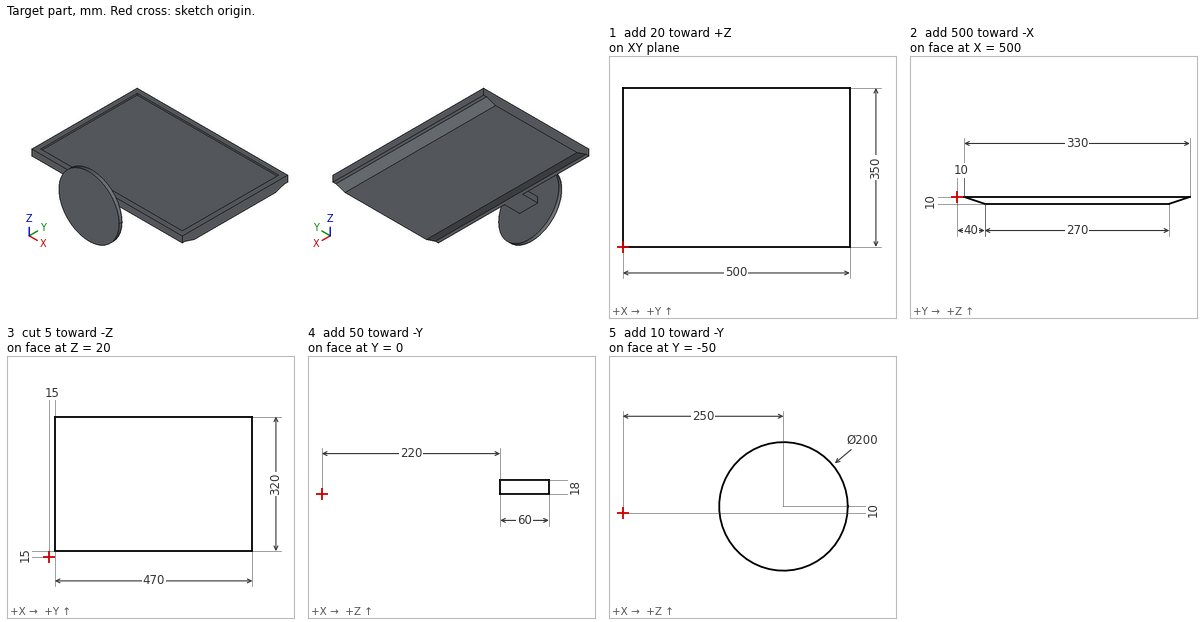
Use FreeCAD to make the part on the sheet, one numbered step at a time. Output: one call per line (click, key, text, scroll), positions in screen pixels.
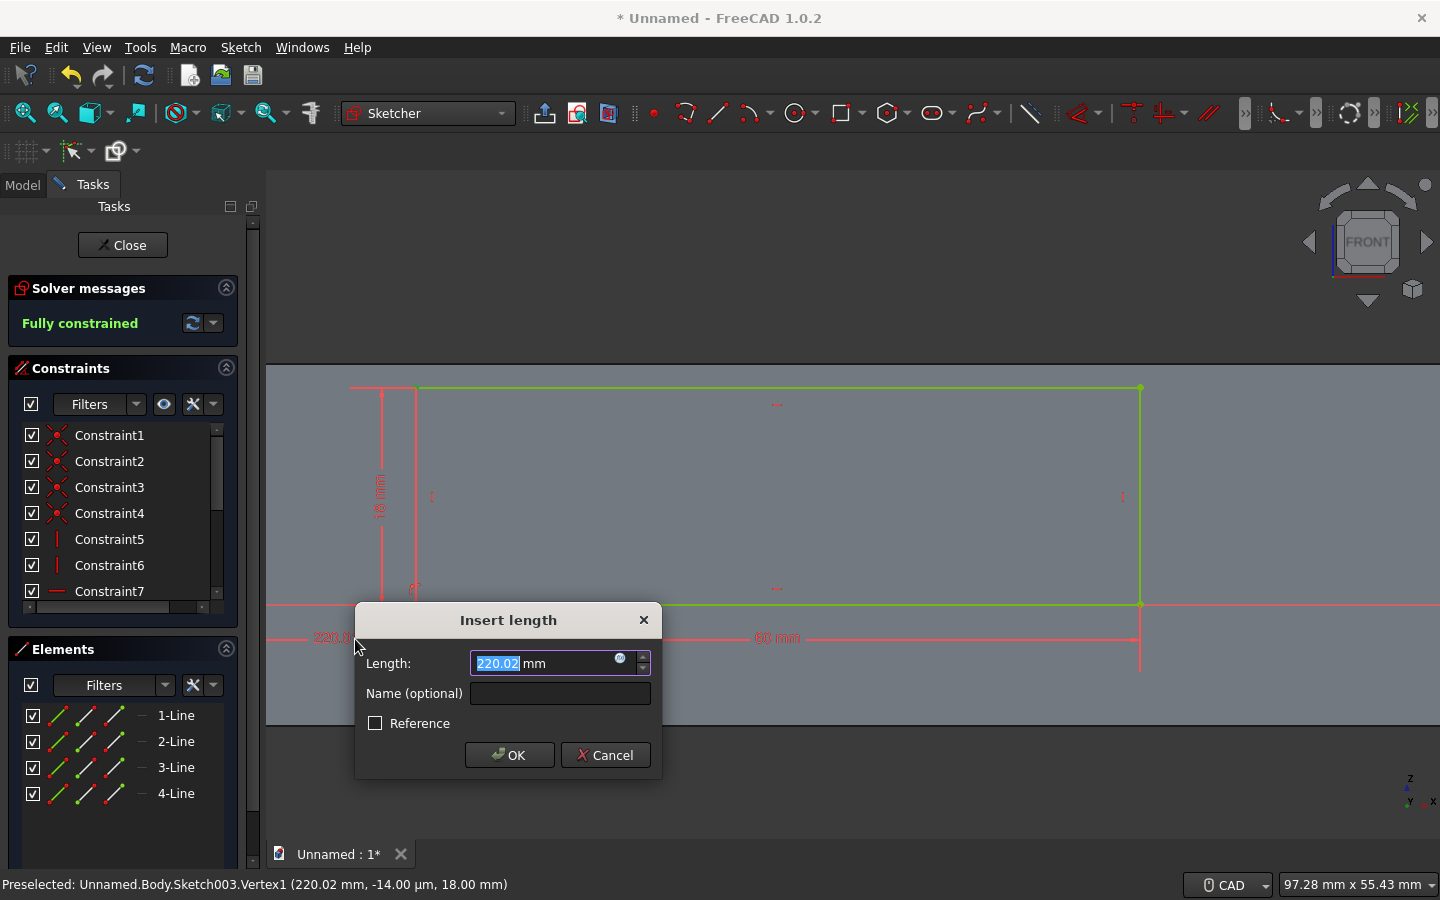
text(220)
key(Return)
key(Escape)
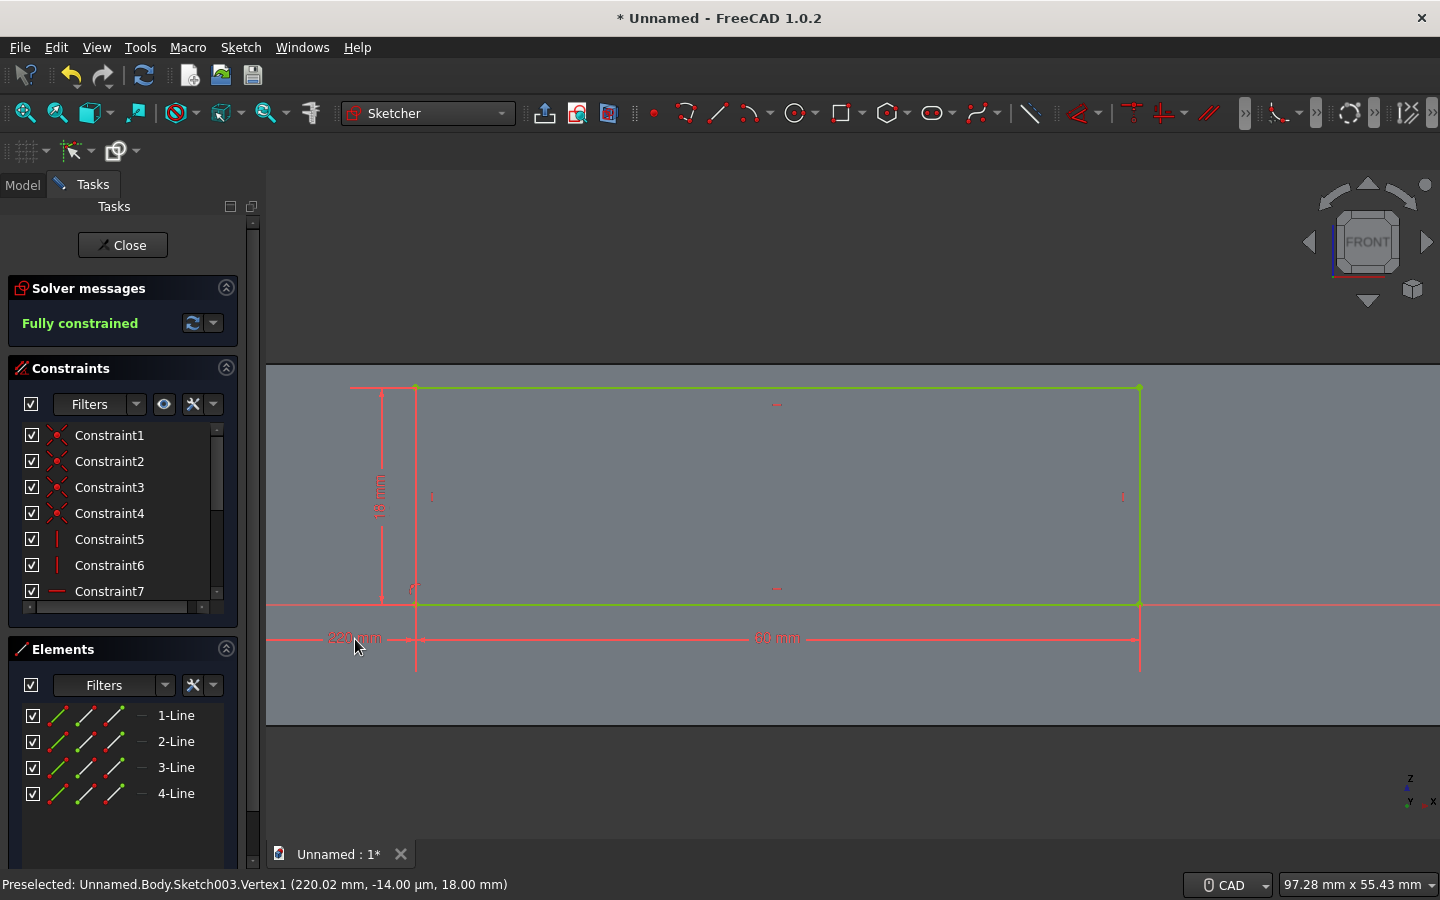
click(123, 245)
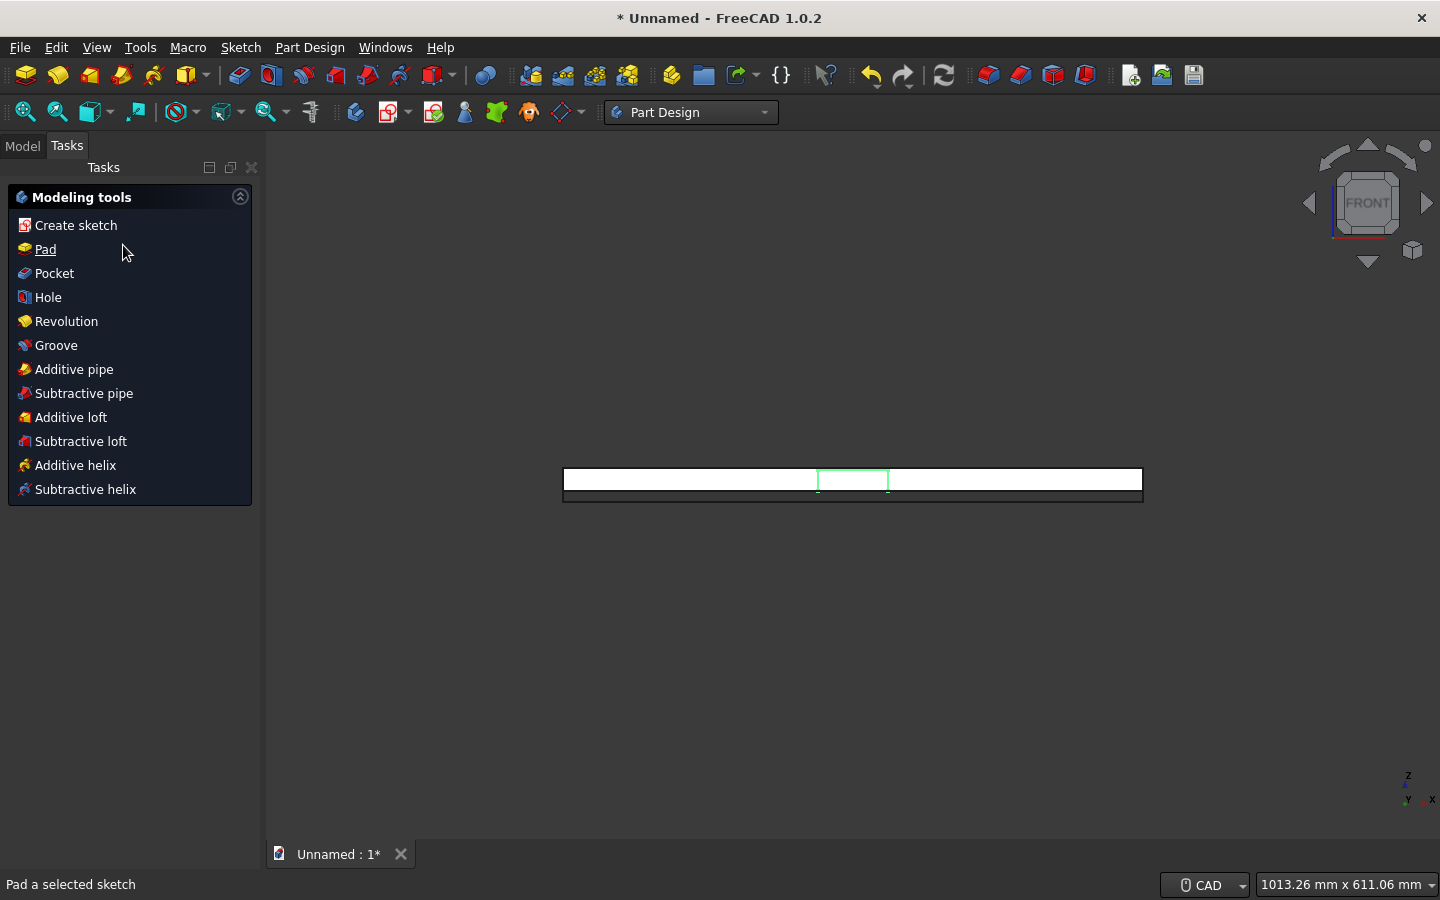
click(26, 76)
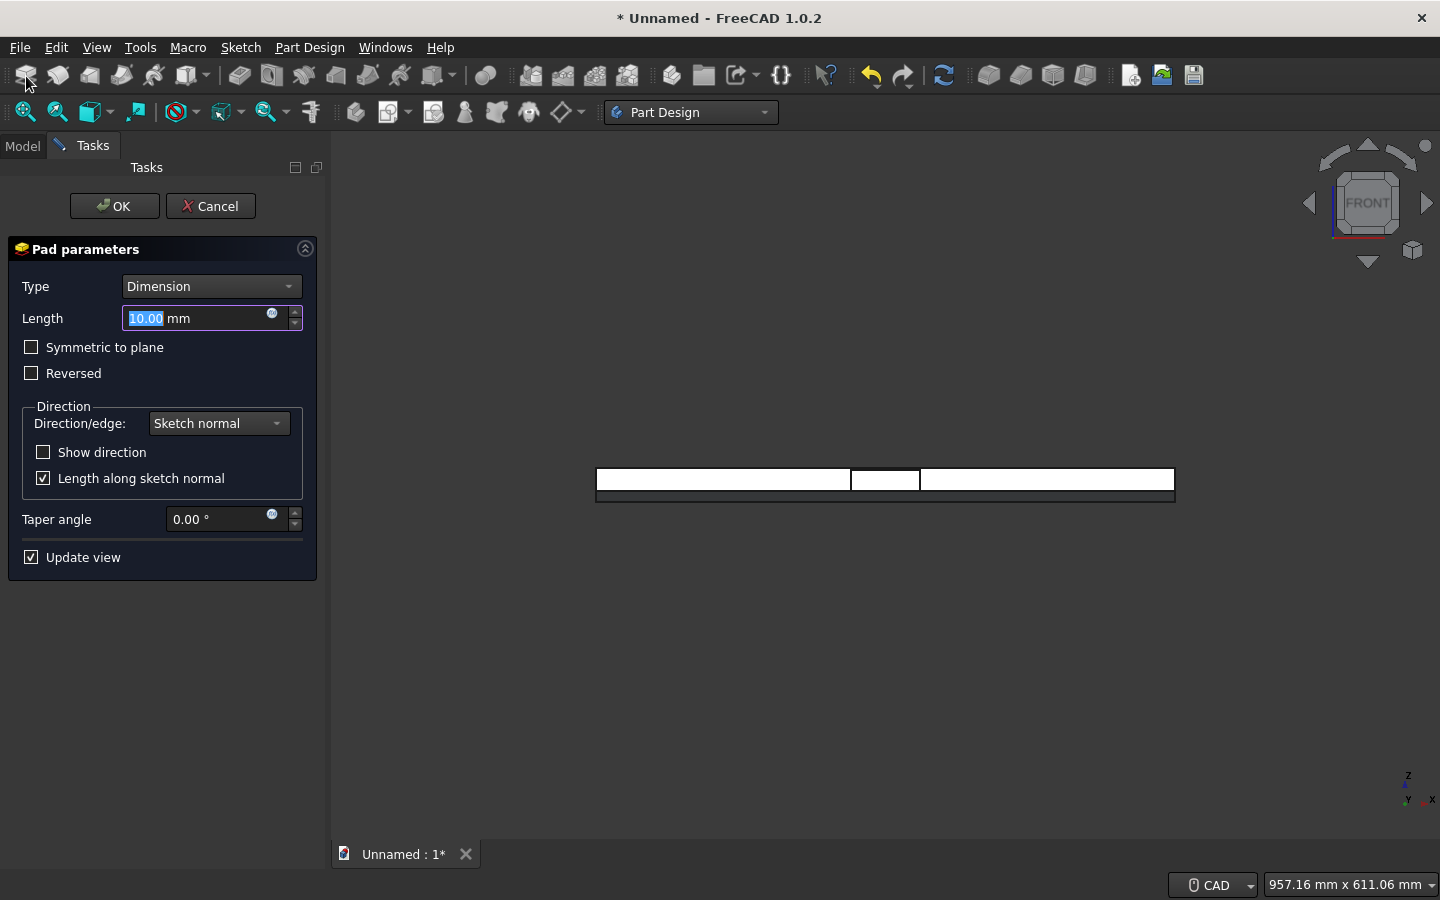
text(50)
key(Tab)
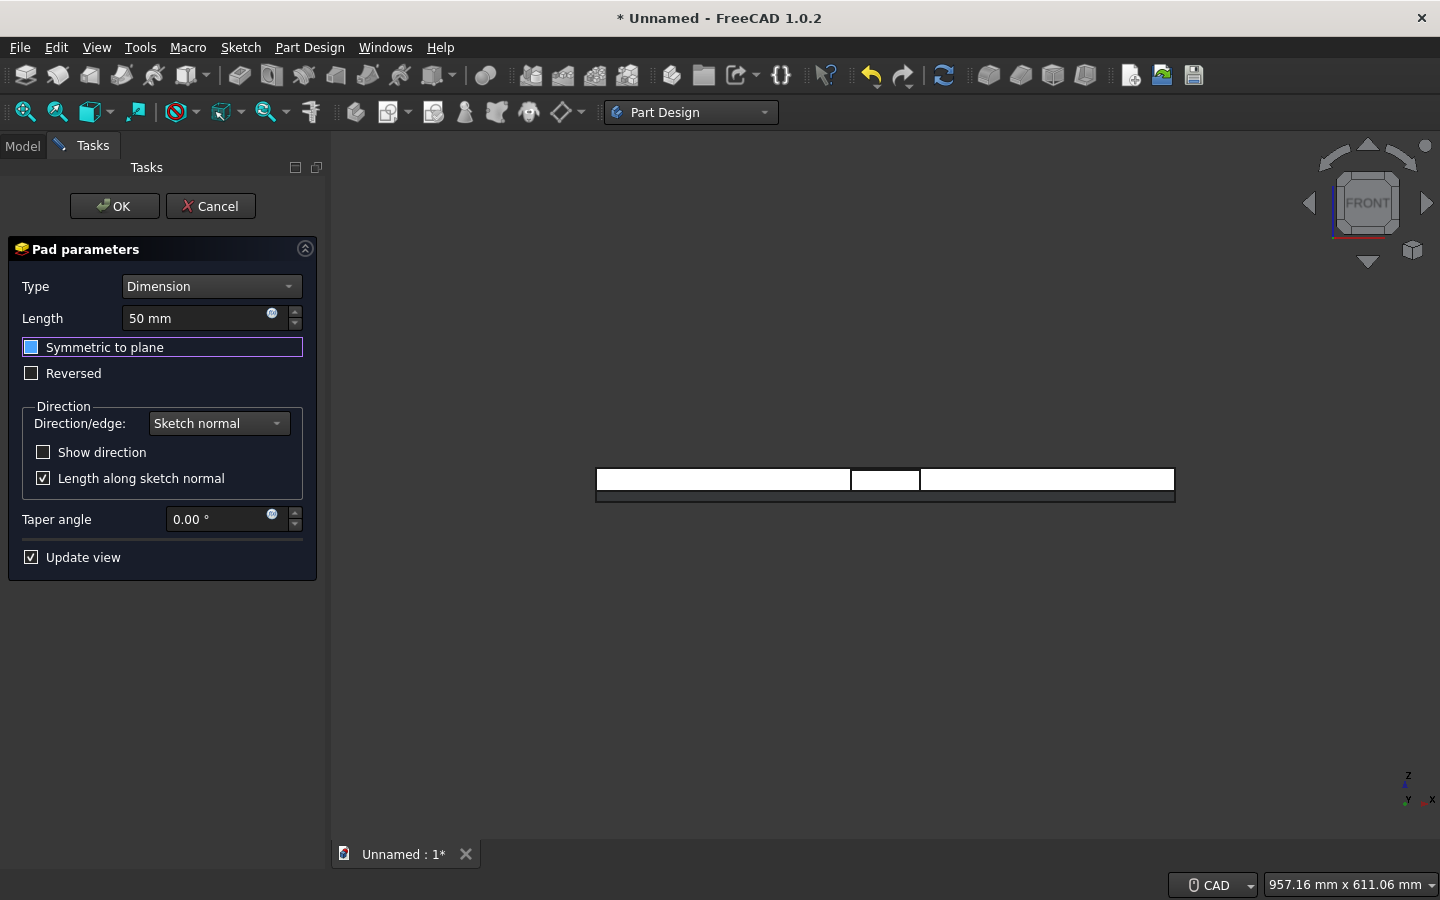
click(115, 206)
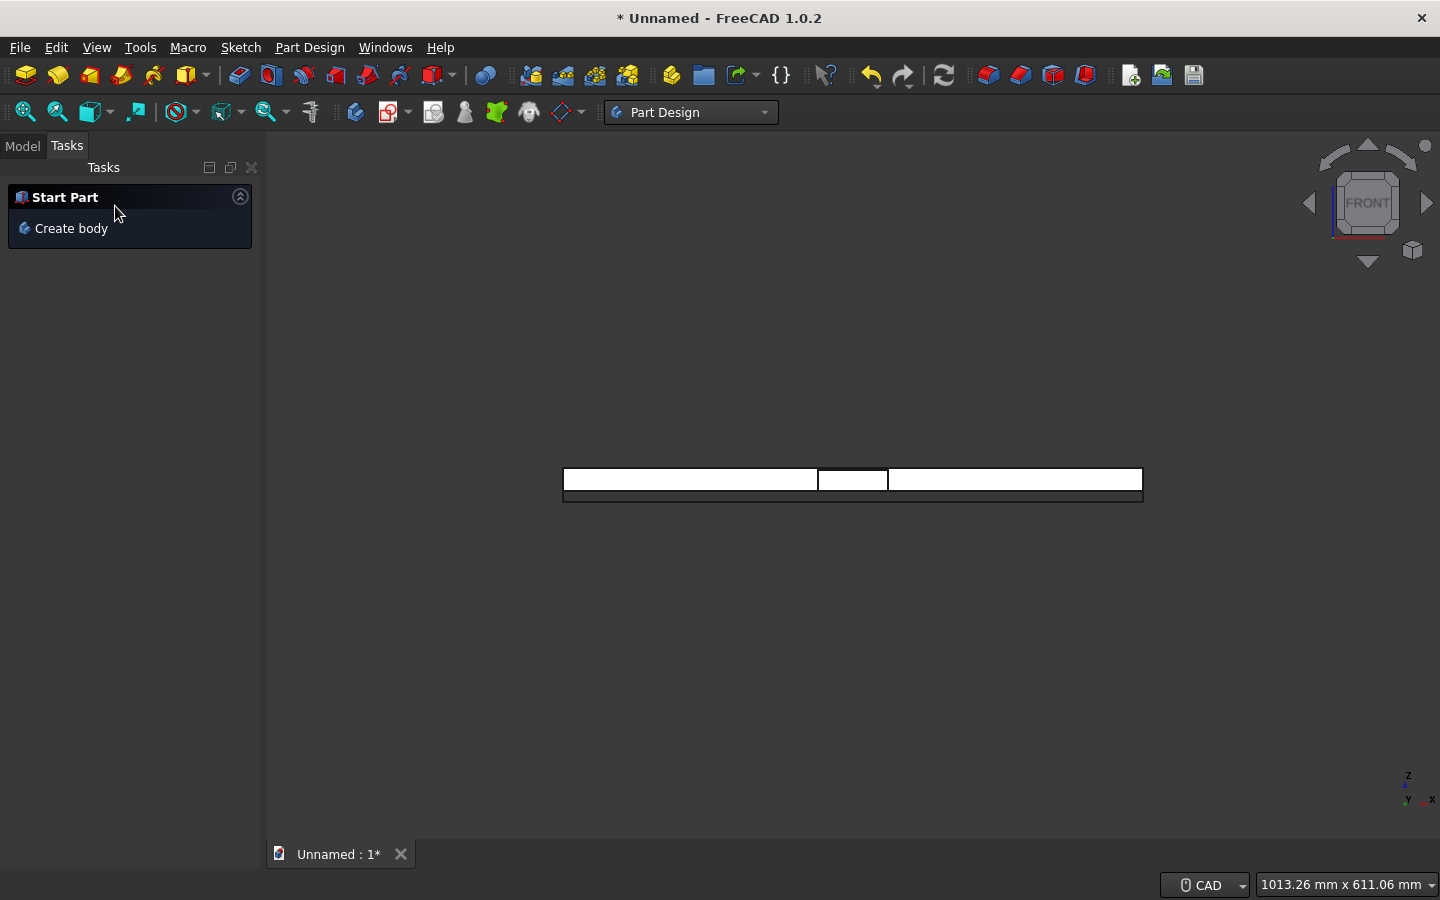
click(873, 479)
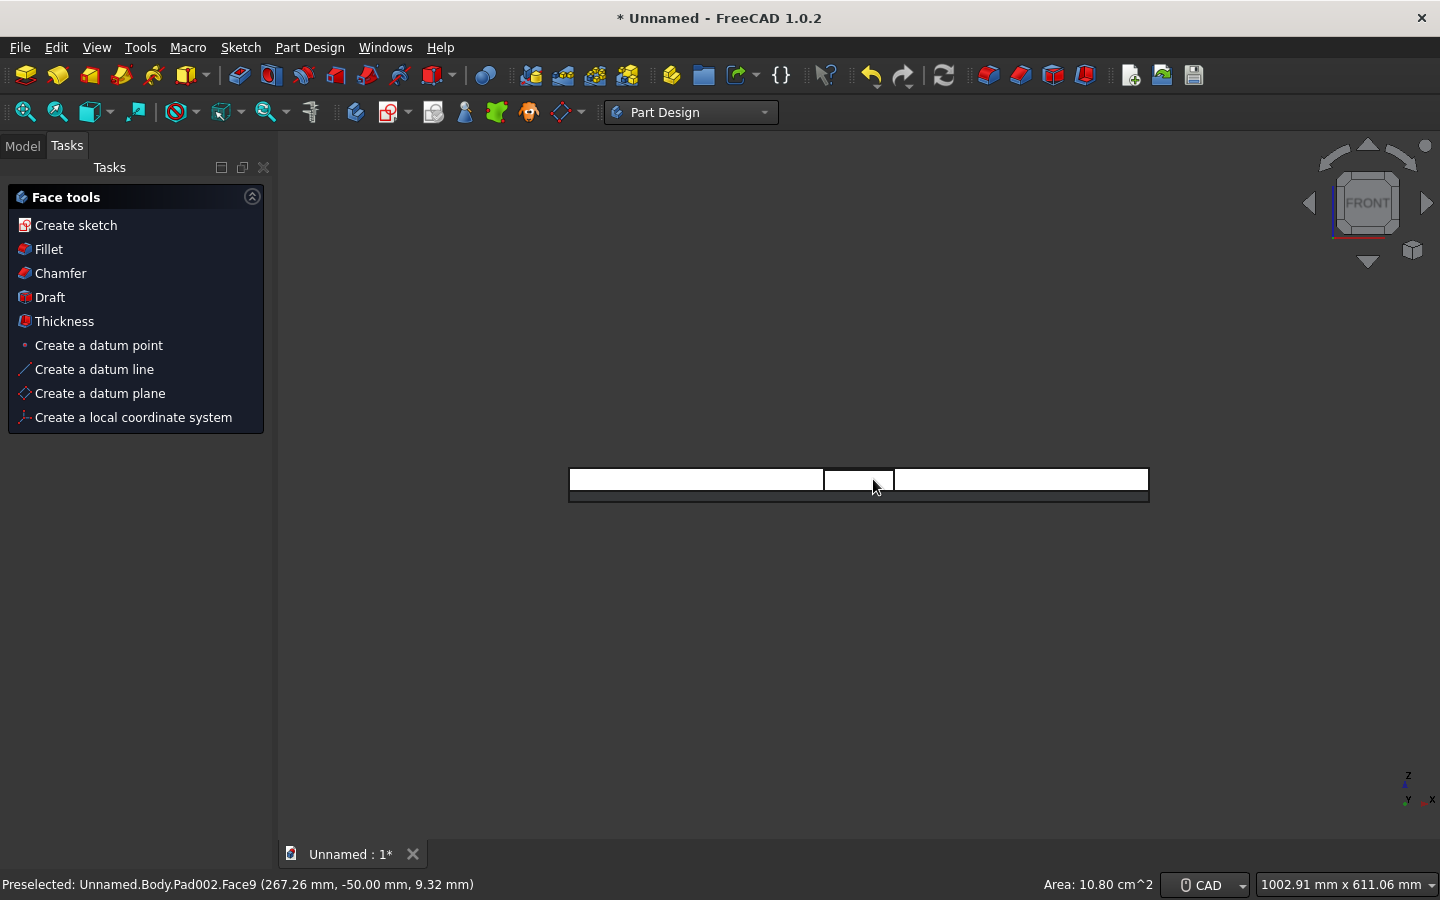
click(388, 112)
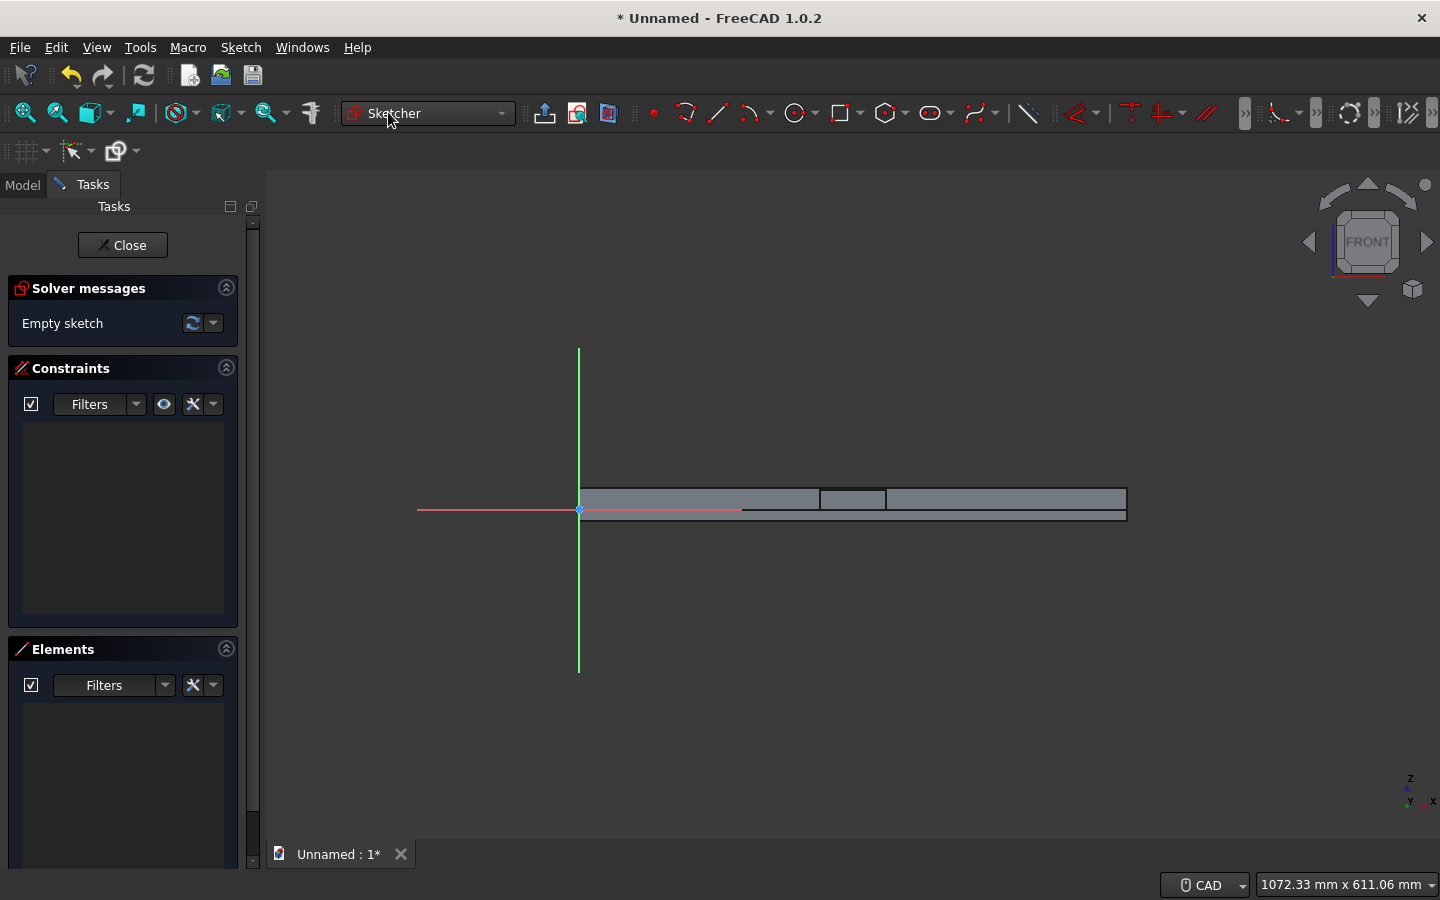
scroll(754, 492, up, 3)